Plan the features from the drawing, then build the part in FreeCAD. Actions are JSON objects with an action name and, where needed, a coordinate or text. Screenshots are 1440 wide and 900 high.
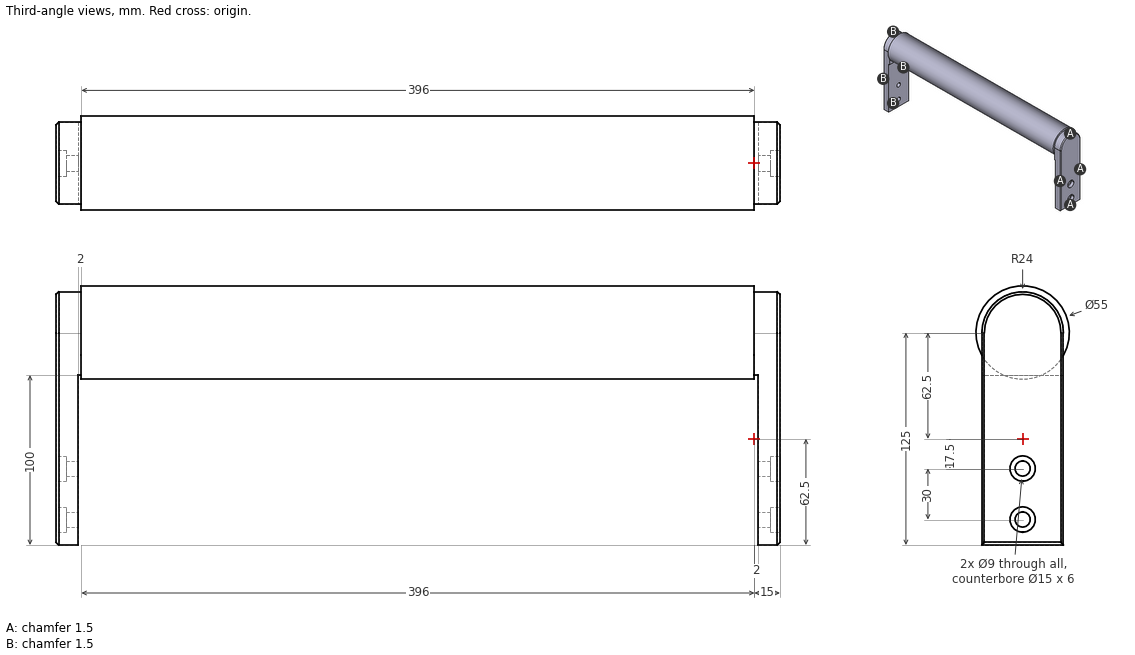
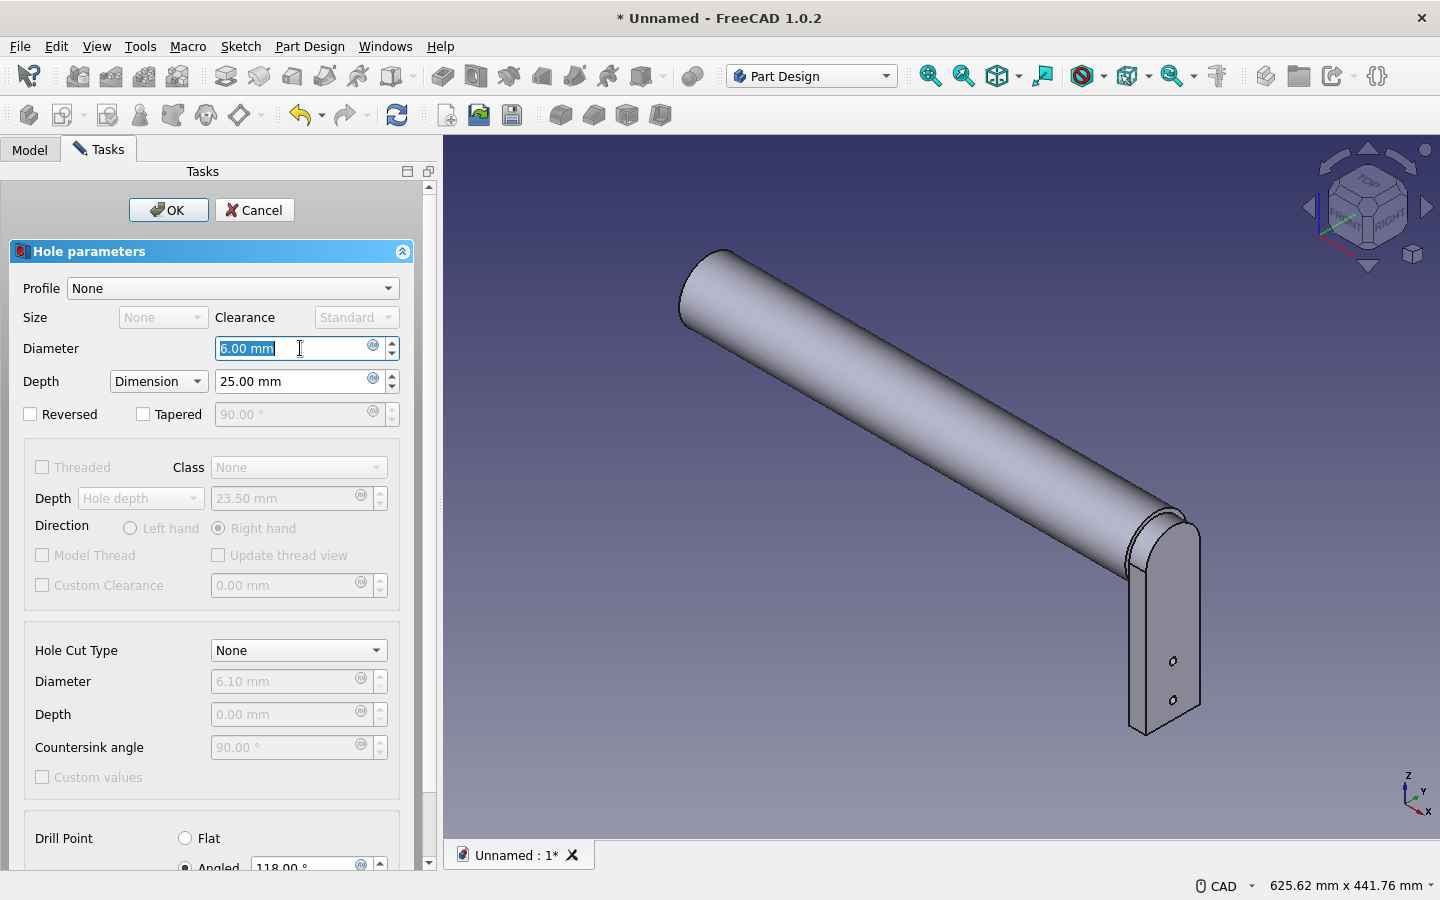
{"action": "type", "text": "9"}
{"action": "key", "text": "Tab"}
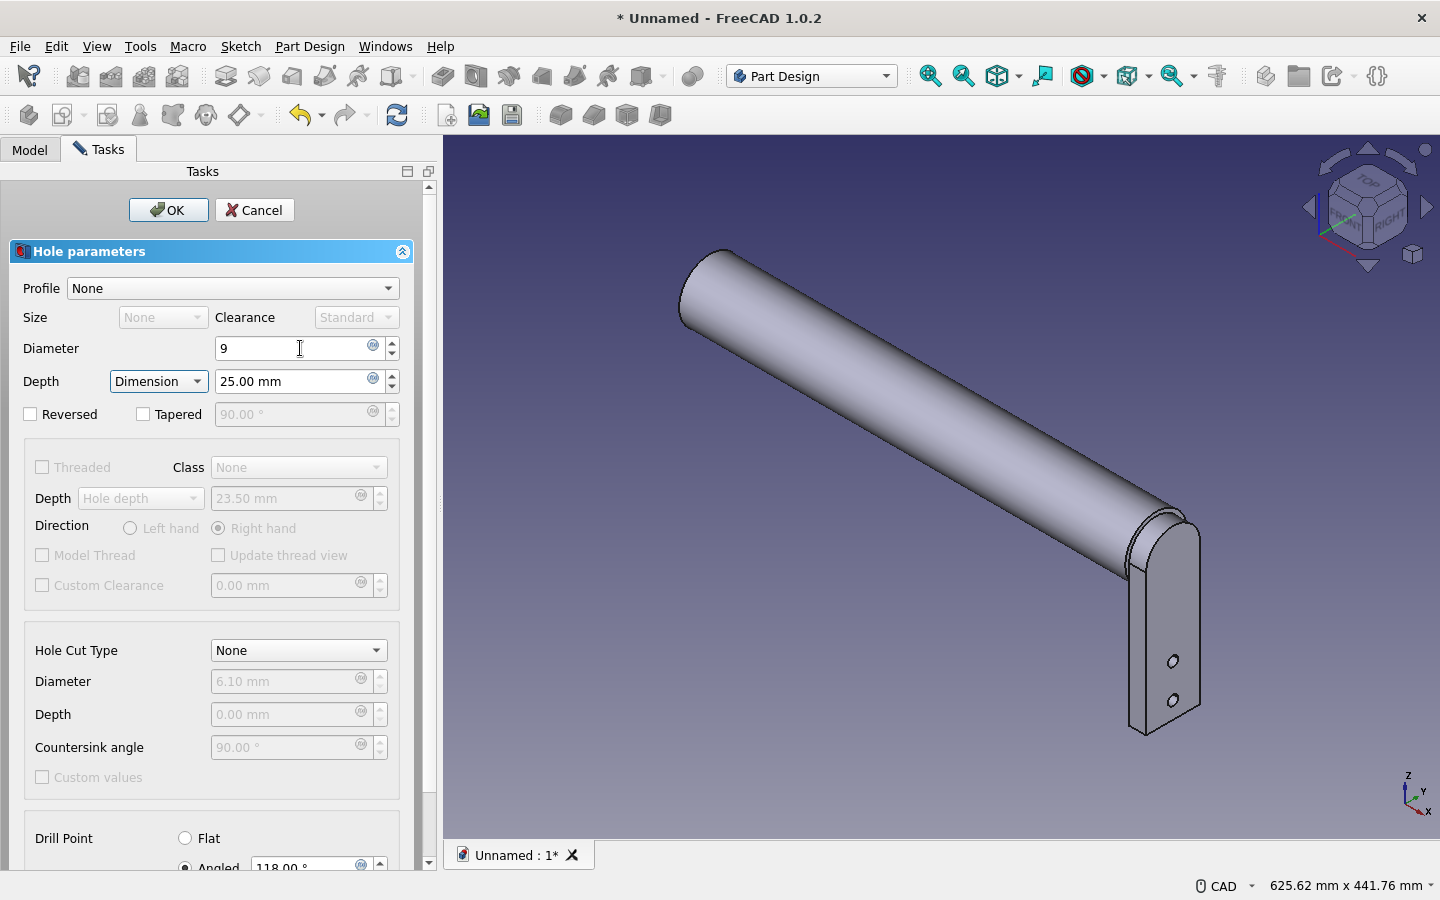
{"action": "left_click", "coordinate": [160, 382]}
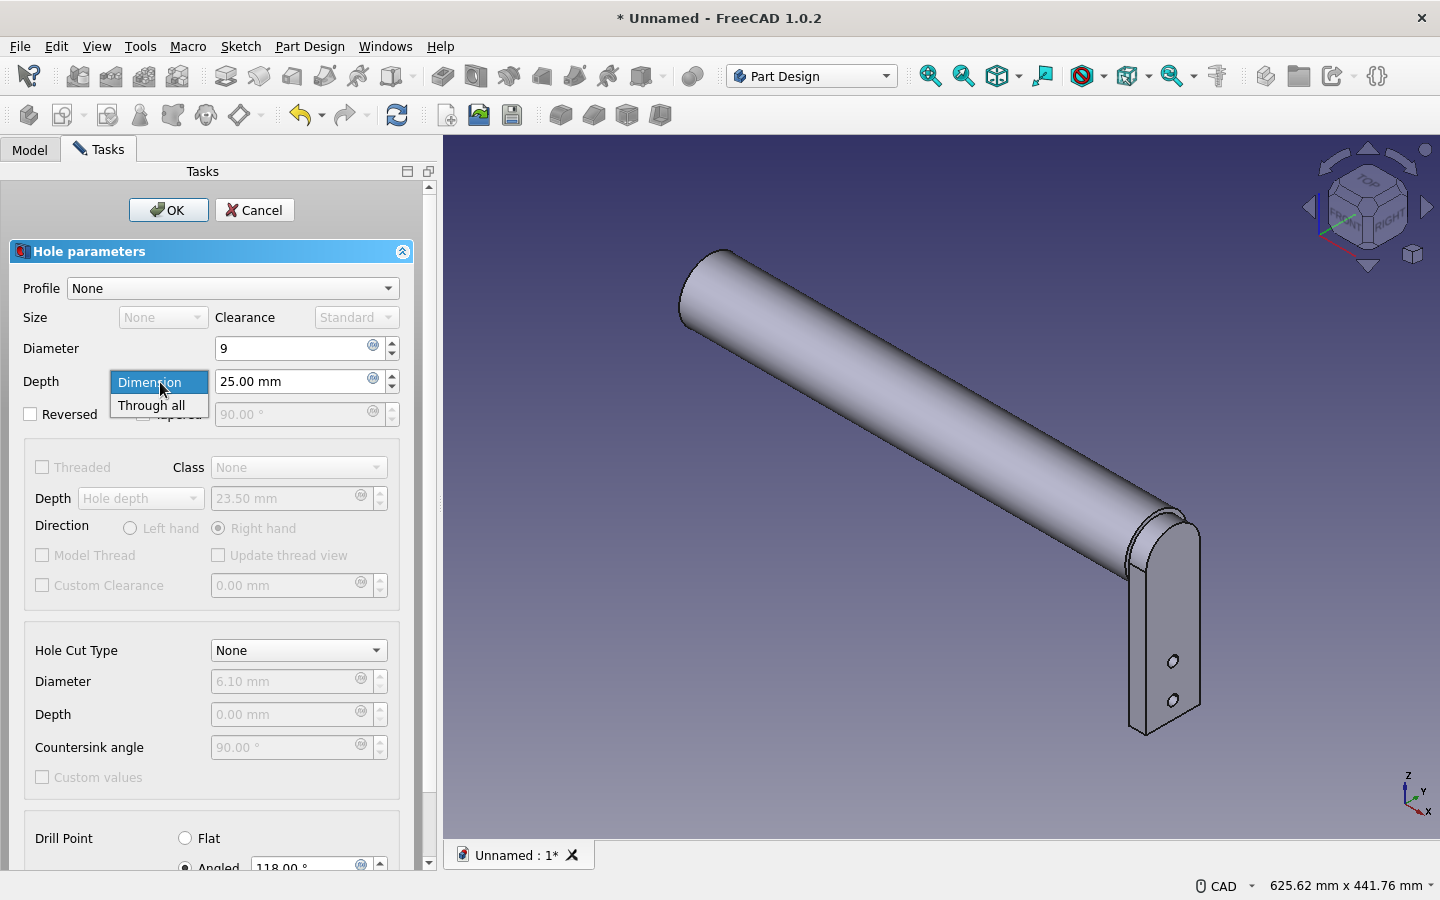
{"action": "left_click", "coordinate": [158, 406]}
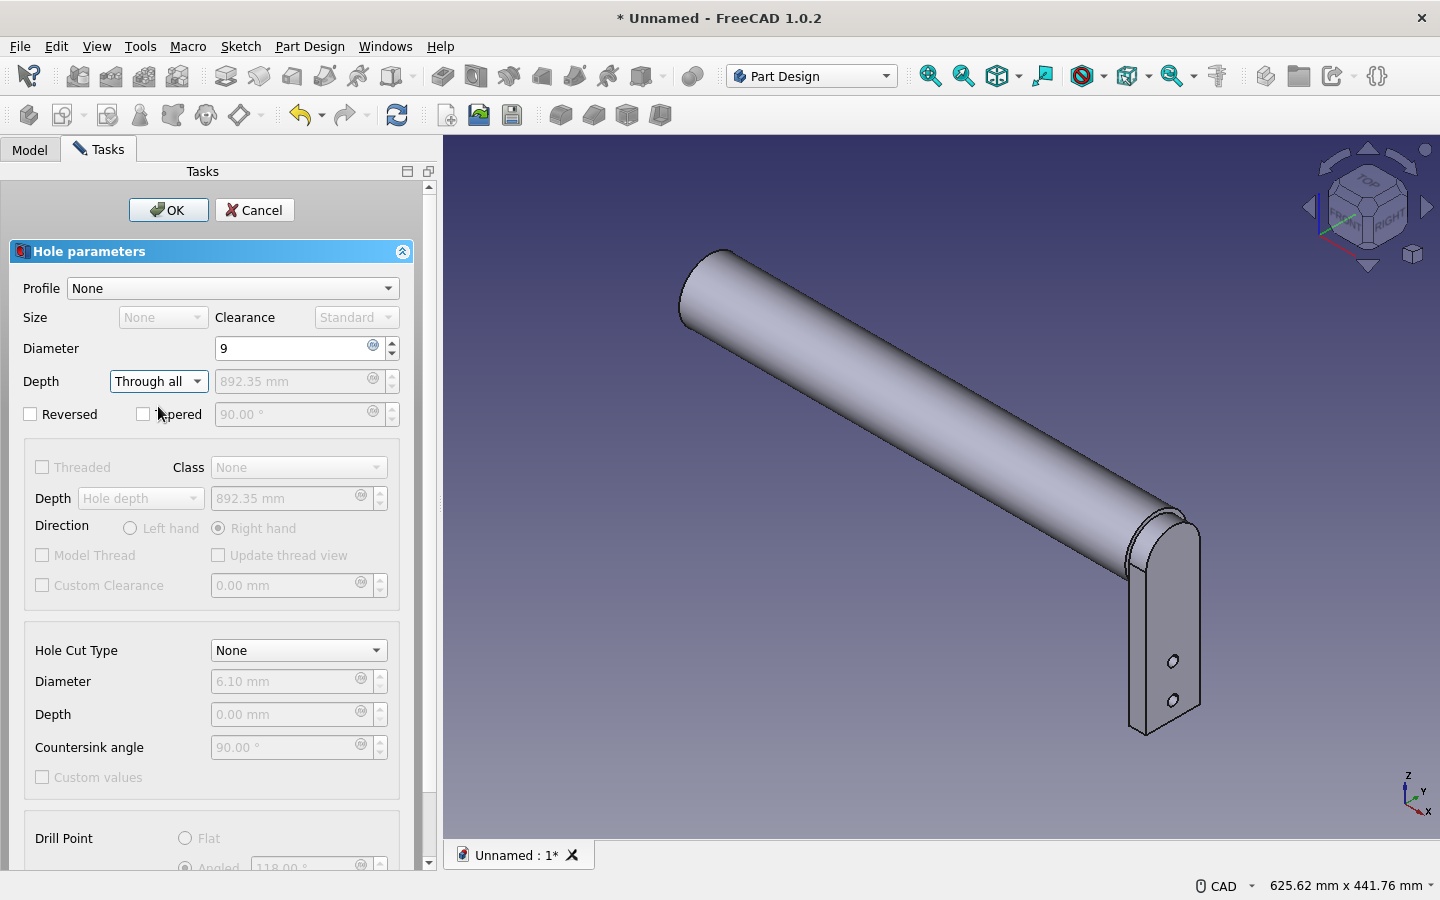
{"action": "left_click", "coordinate": [300, 650]}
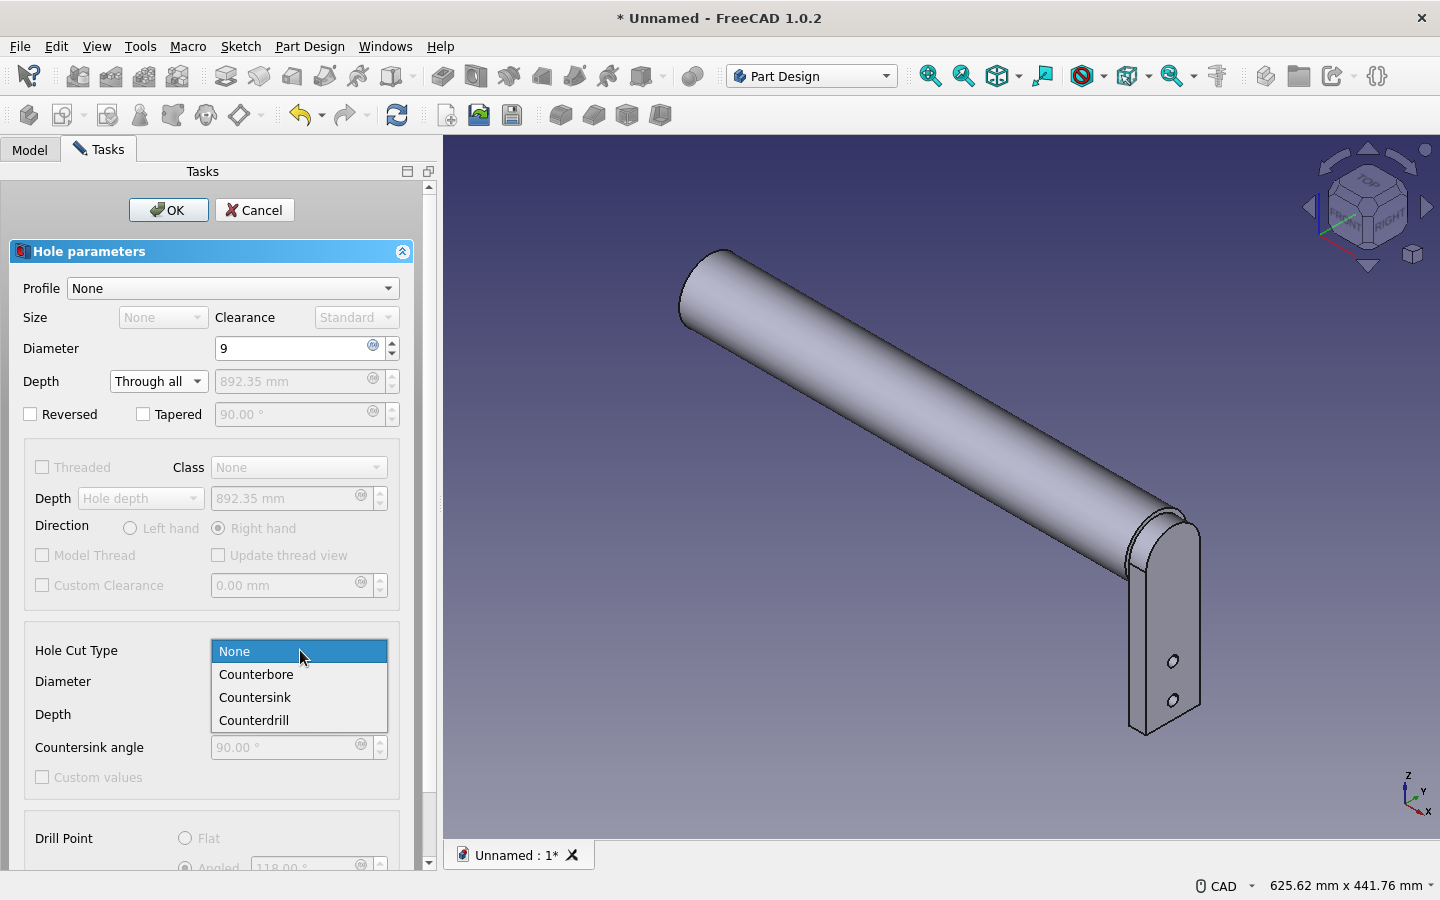
{"action": "left_click", "coordinate": [298, 674]}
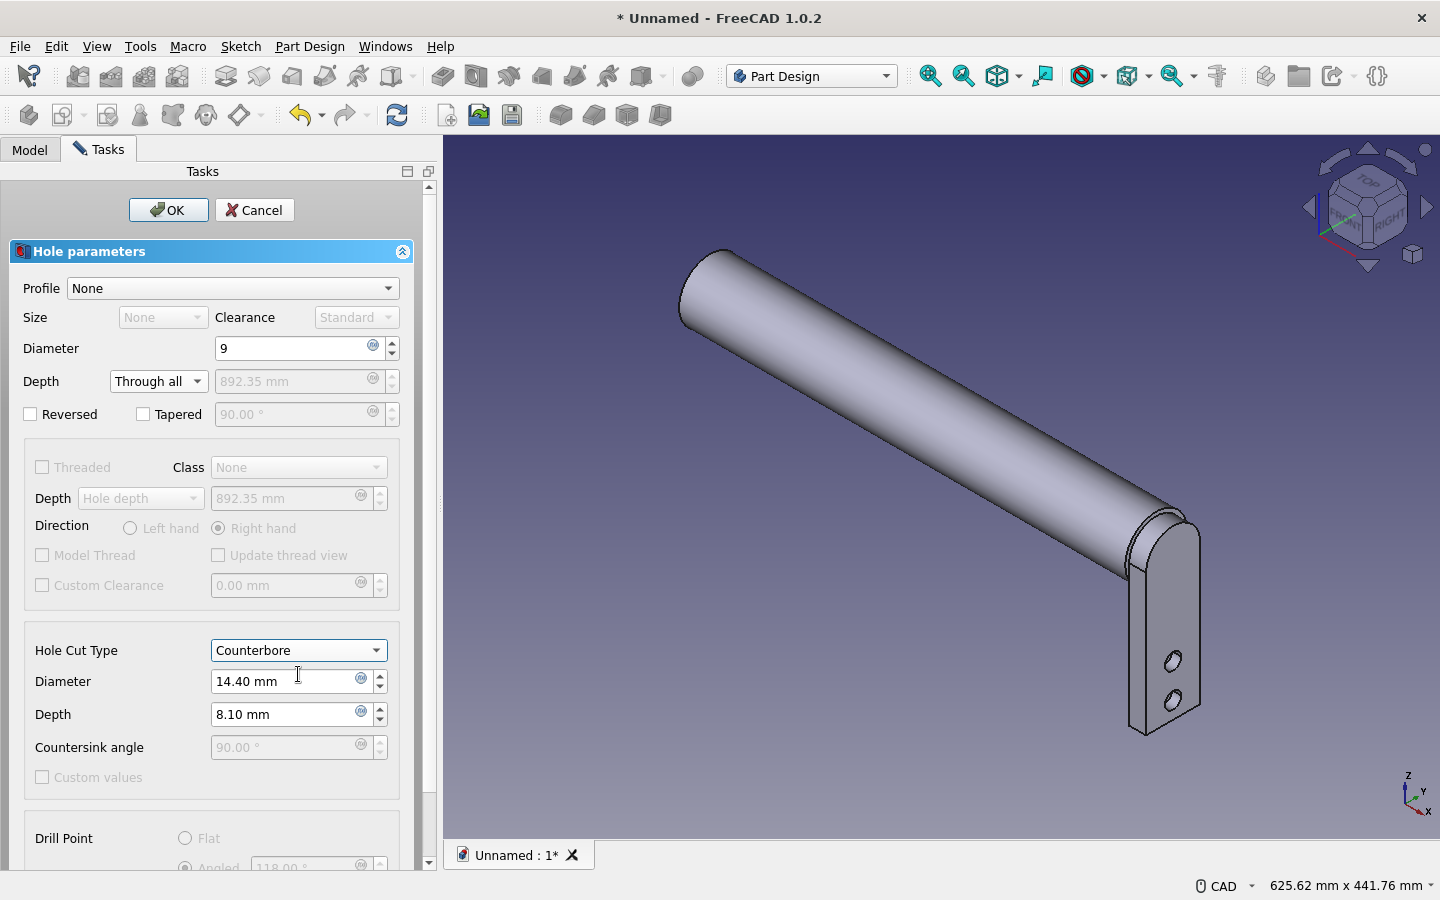
{"action": "triple_click", "coordinate": [292, 682]}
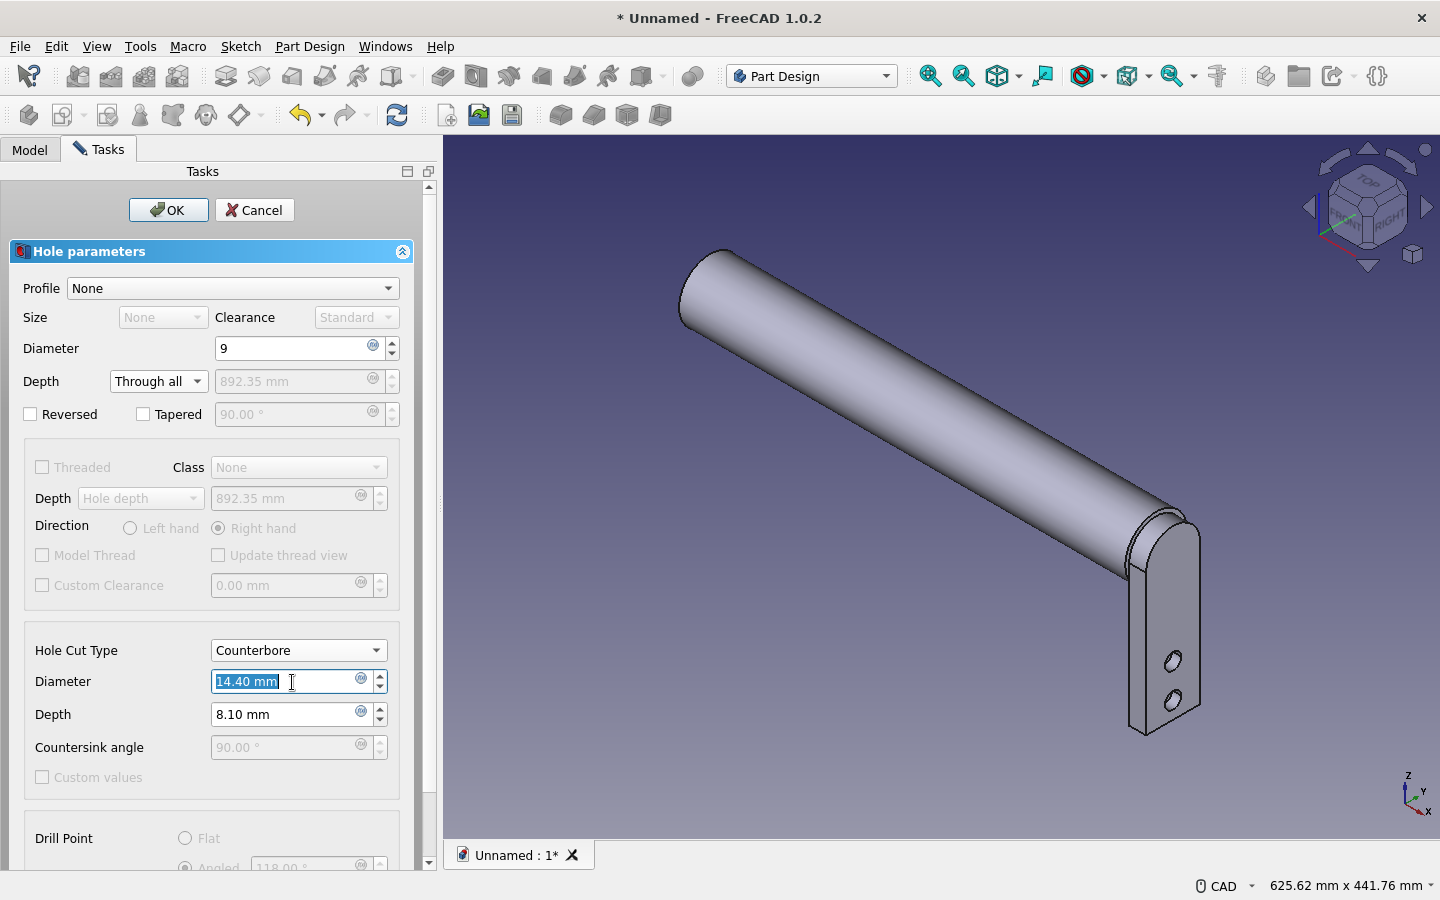
{"action": "type", "text": "15"}
{"action": "key", "text": "Tab"}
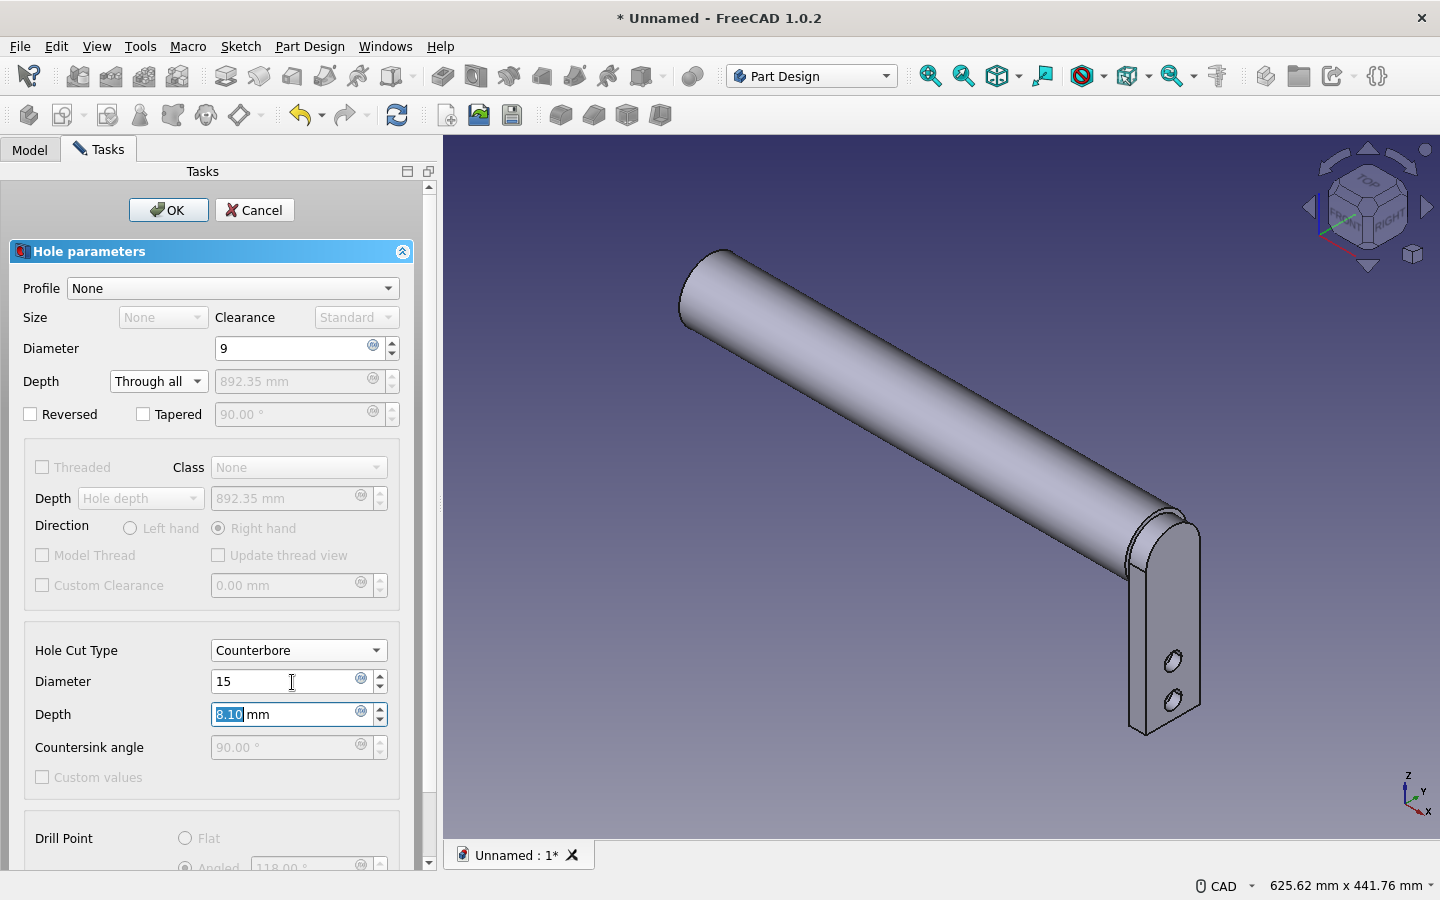
{"action": "type", "text": "6"}
{"action": "key", "text": "Tab"}